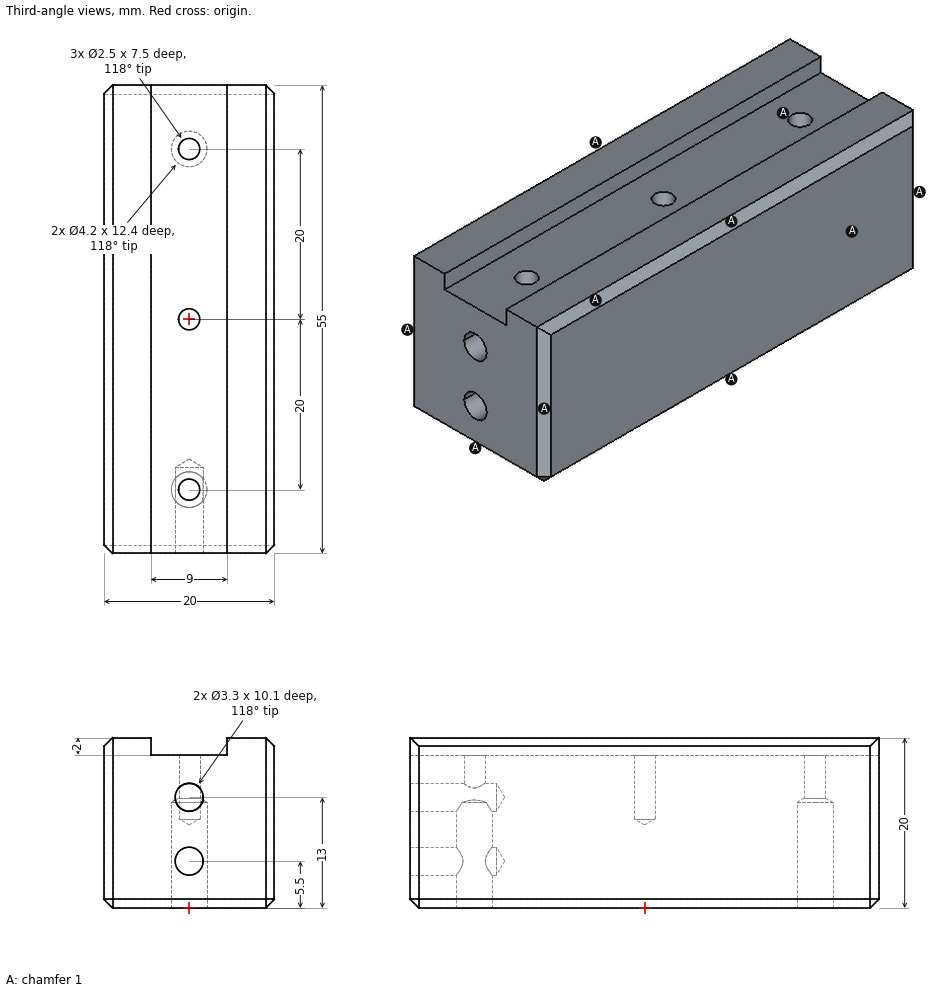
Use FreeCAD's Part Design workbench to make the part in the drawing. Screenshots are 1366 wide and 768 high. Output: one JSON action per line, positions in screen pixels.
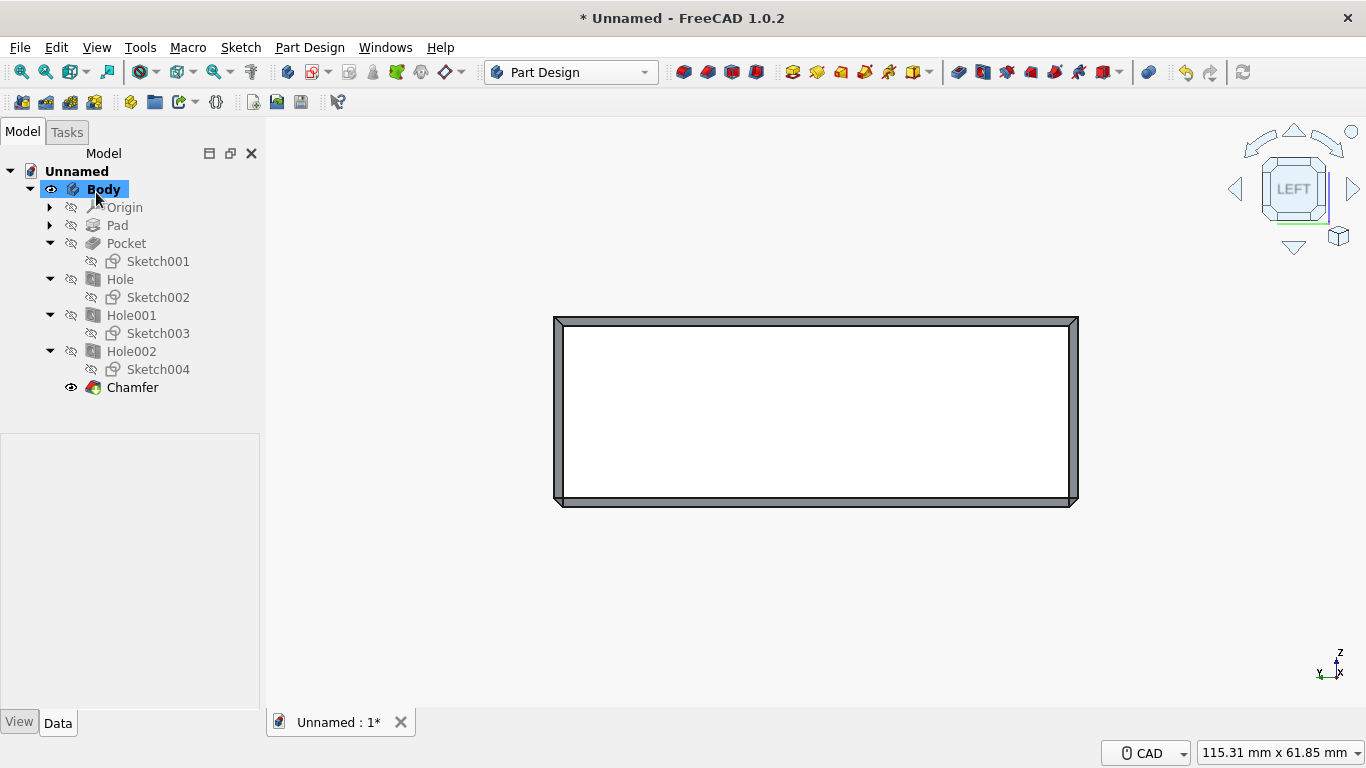
{"action": "key", "text": "0"}